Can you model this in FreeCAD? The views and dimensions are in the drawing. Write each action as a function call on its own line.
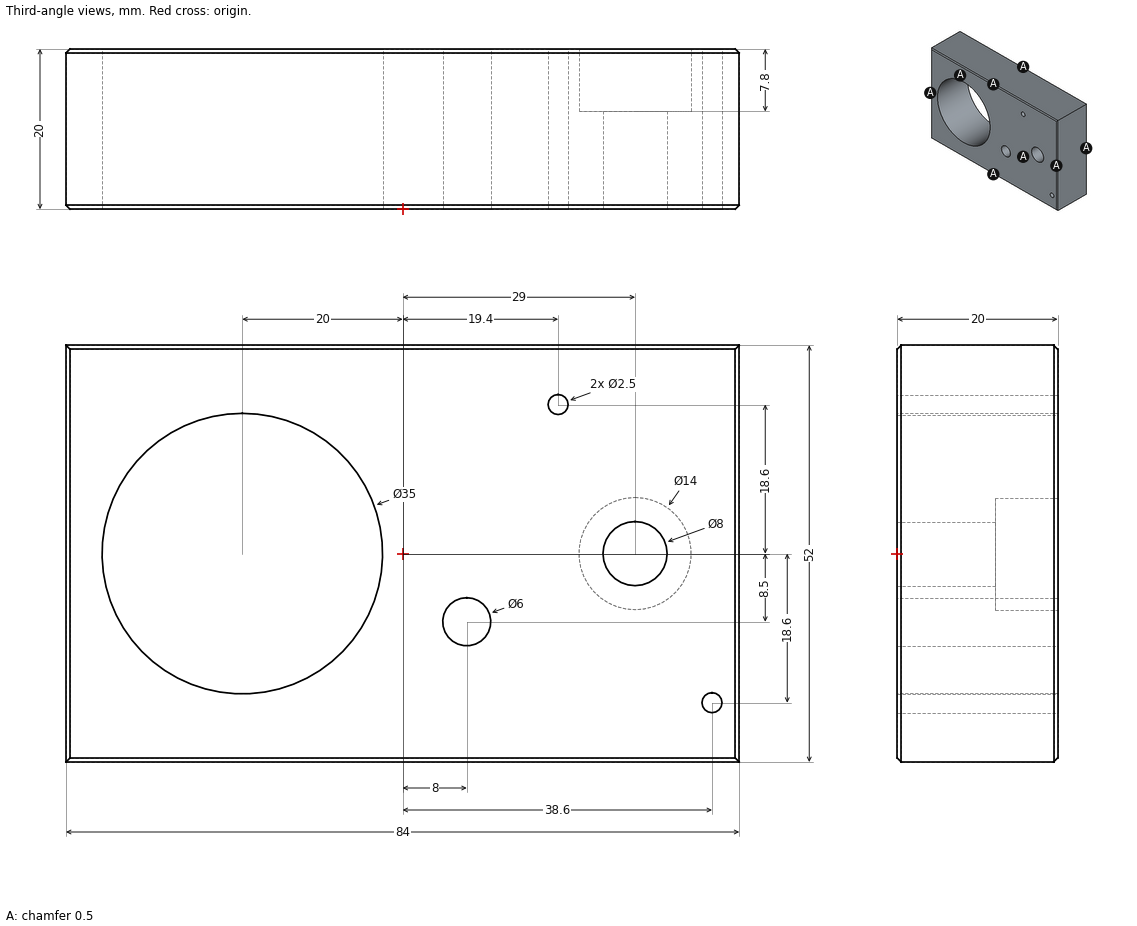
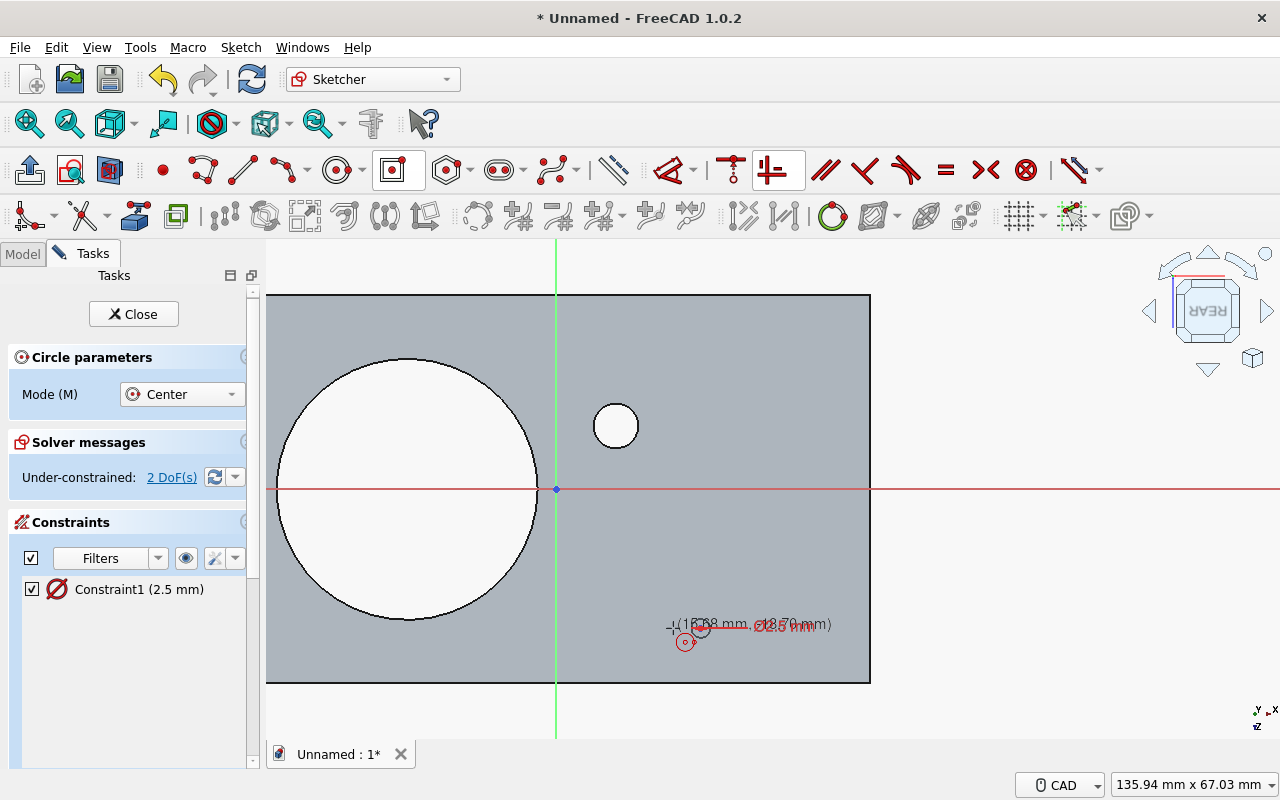
scroll(844, 351, up, 5)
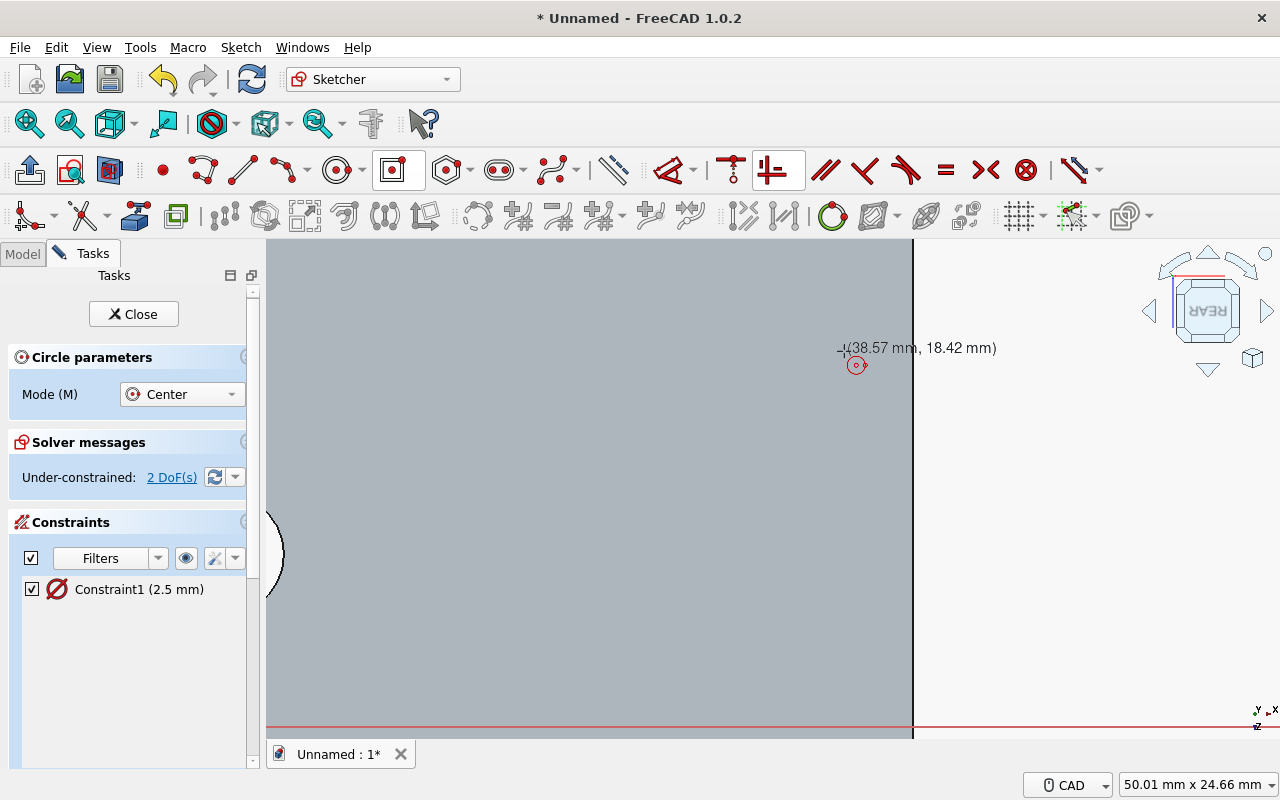
click(844, 350)
move(862, 332)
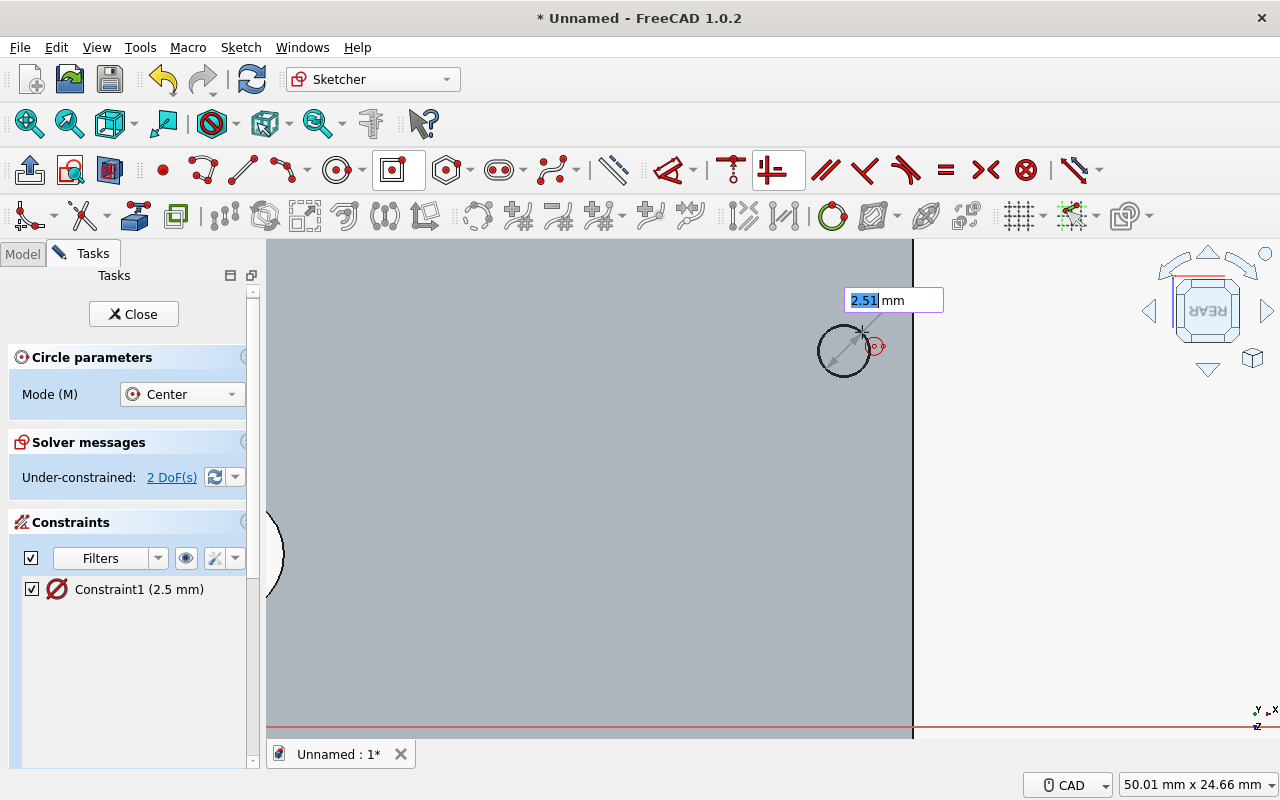
text(2.5)
key(Return)
key(Escape)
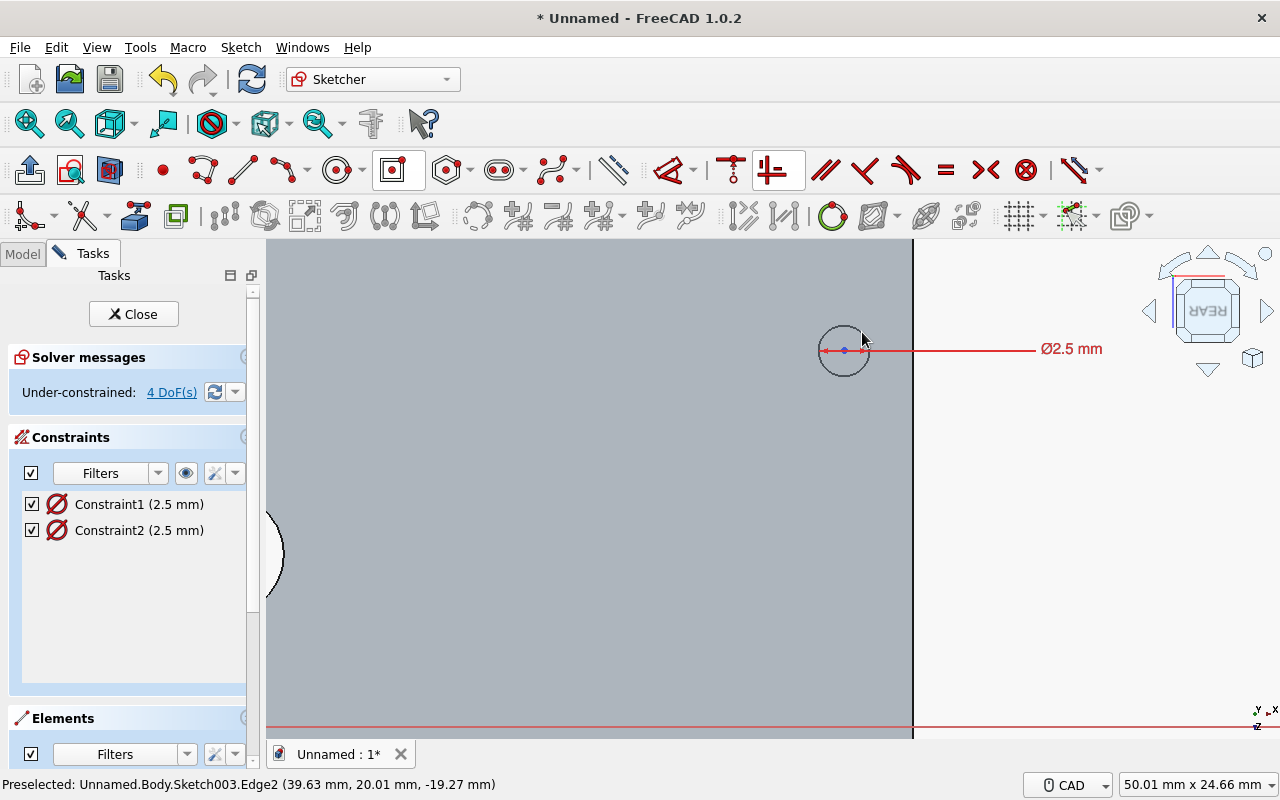
click(668, 170)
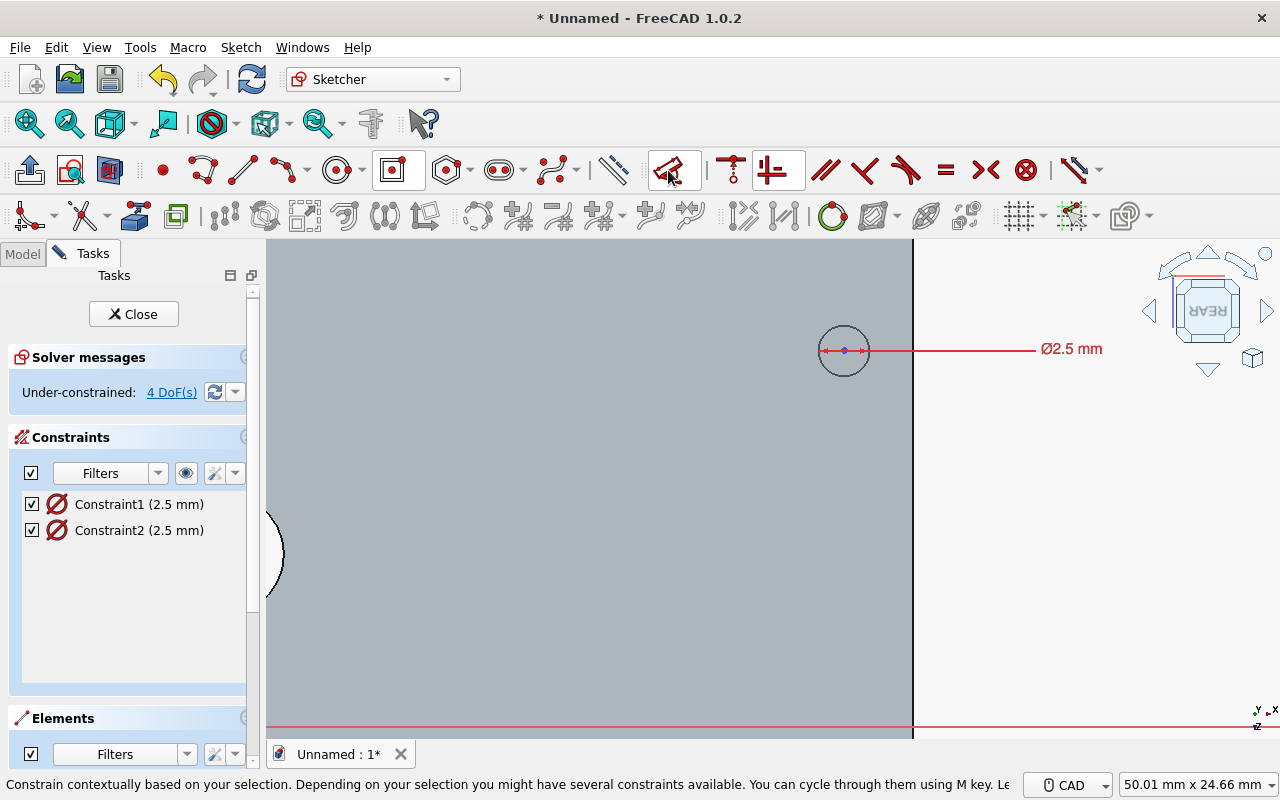
scroll(844, 351, down, 5)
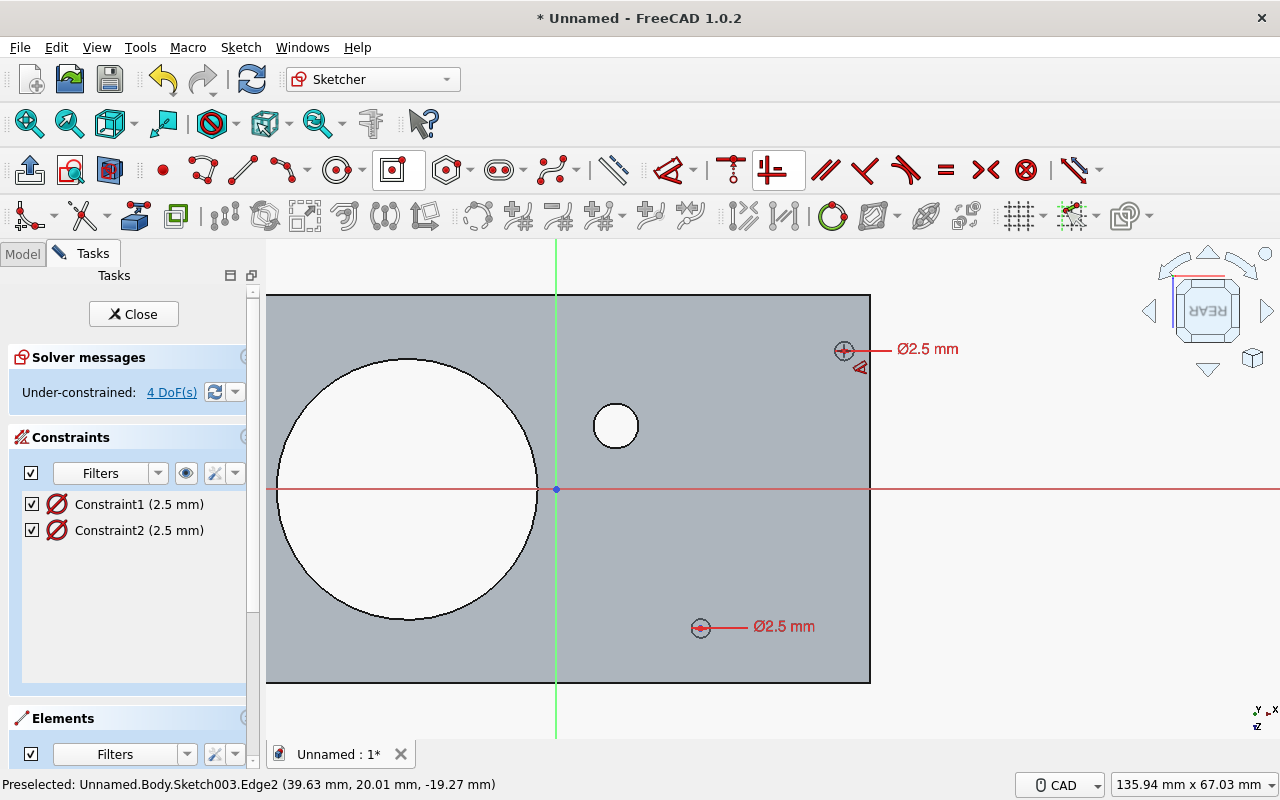
click(701, 628)
click(629, 662)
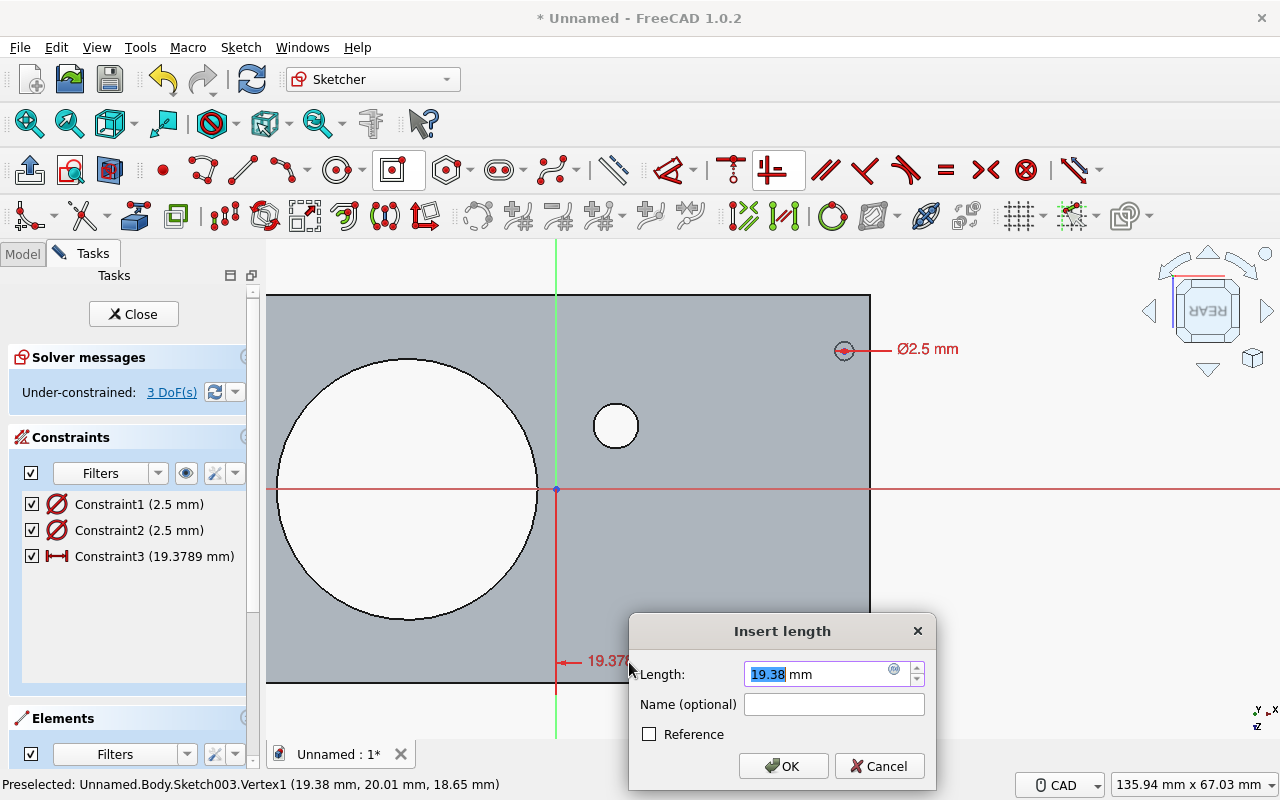
text(19.4)
key(Return)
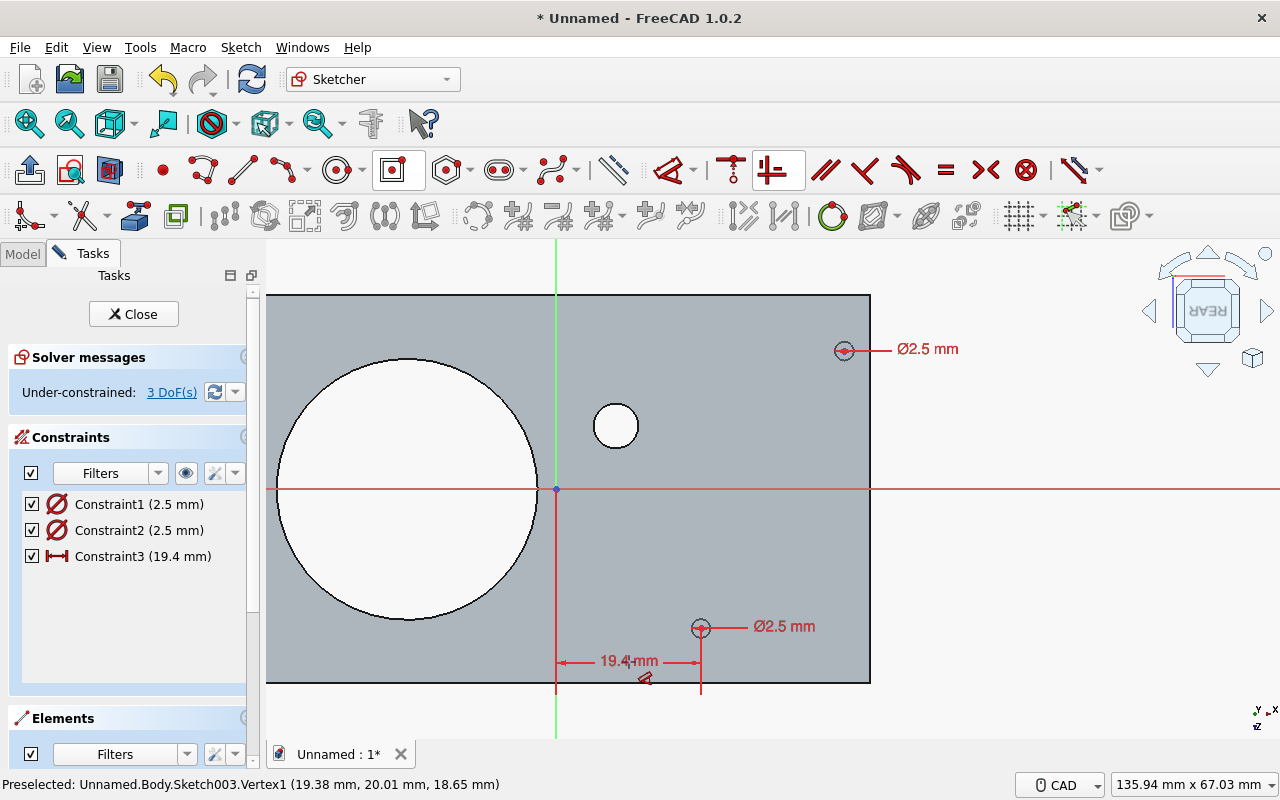
click(701, 628)
click(522, 559)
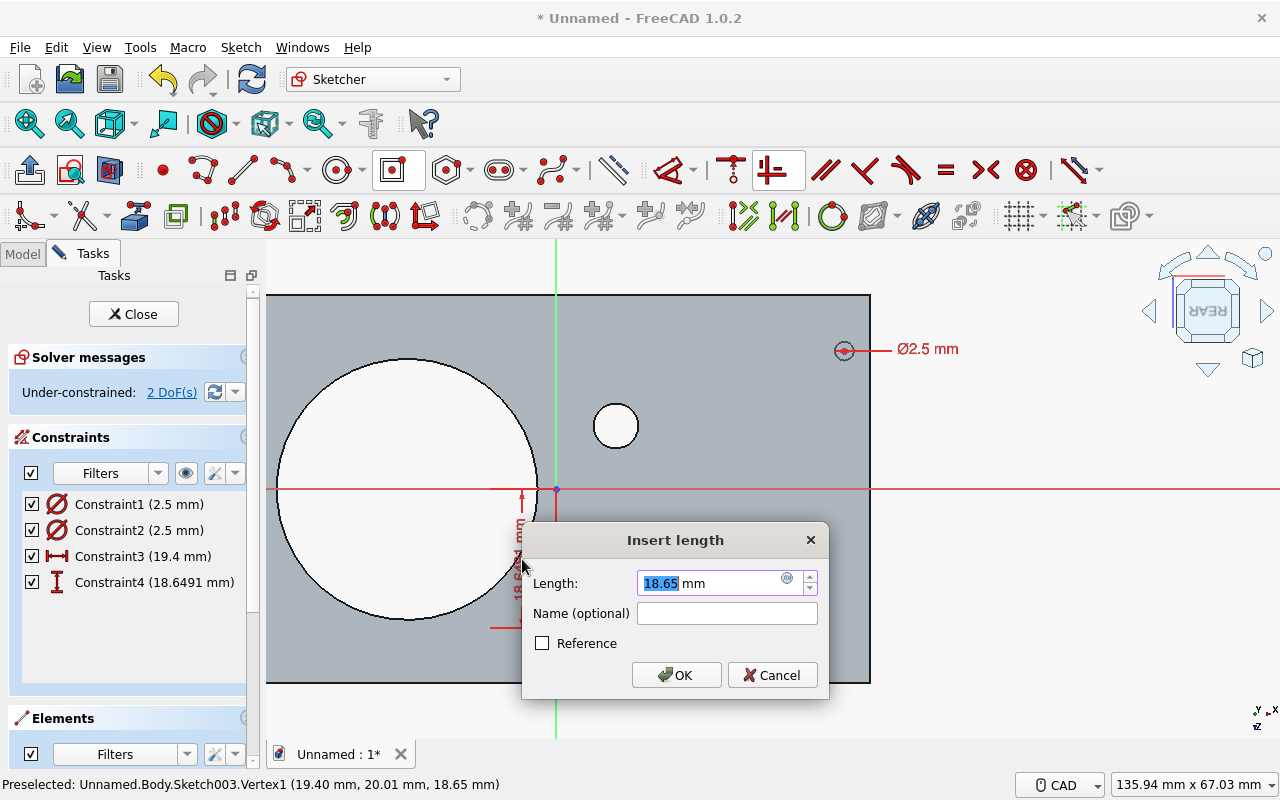
text(18.6)
key(Return)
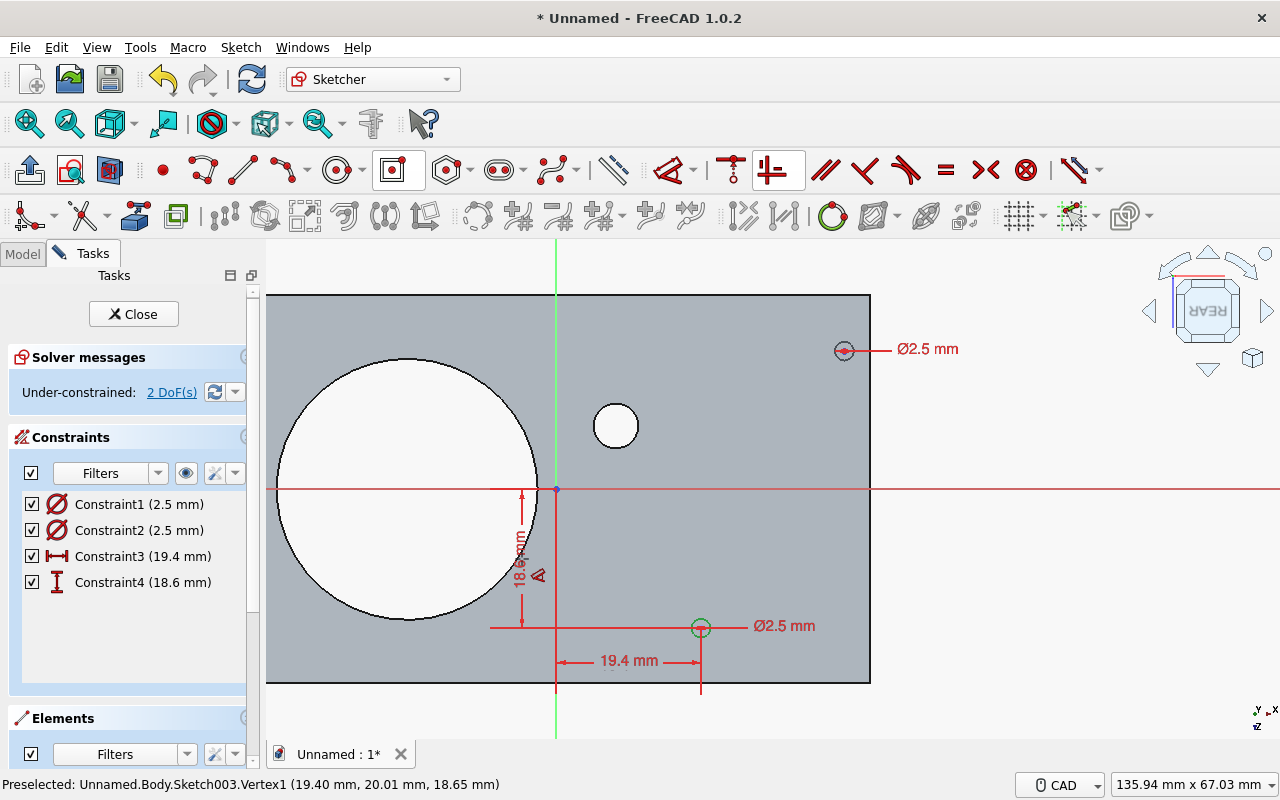
click(844, 351)
click(700, 317)